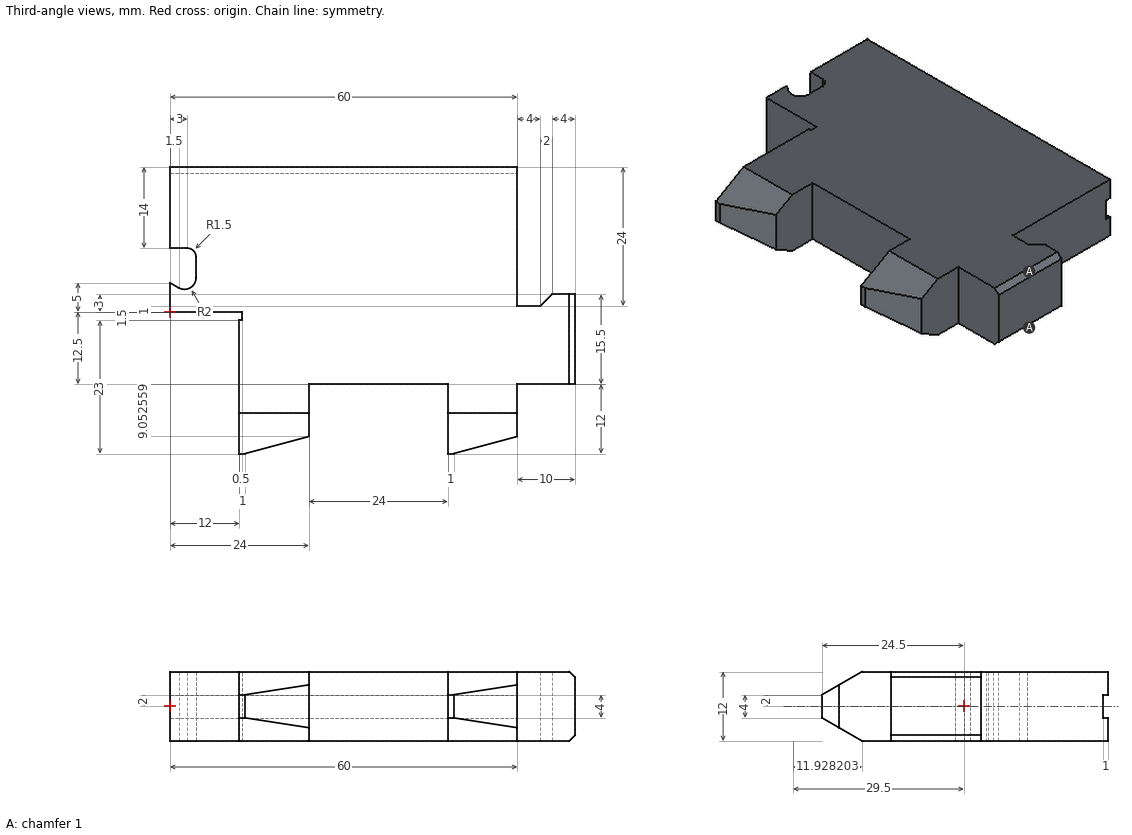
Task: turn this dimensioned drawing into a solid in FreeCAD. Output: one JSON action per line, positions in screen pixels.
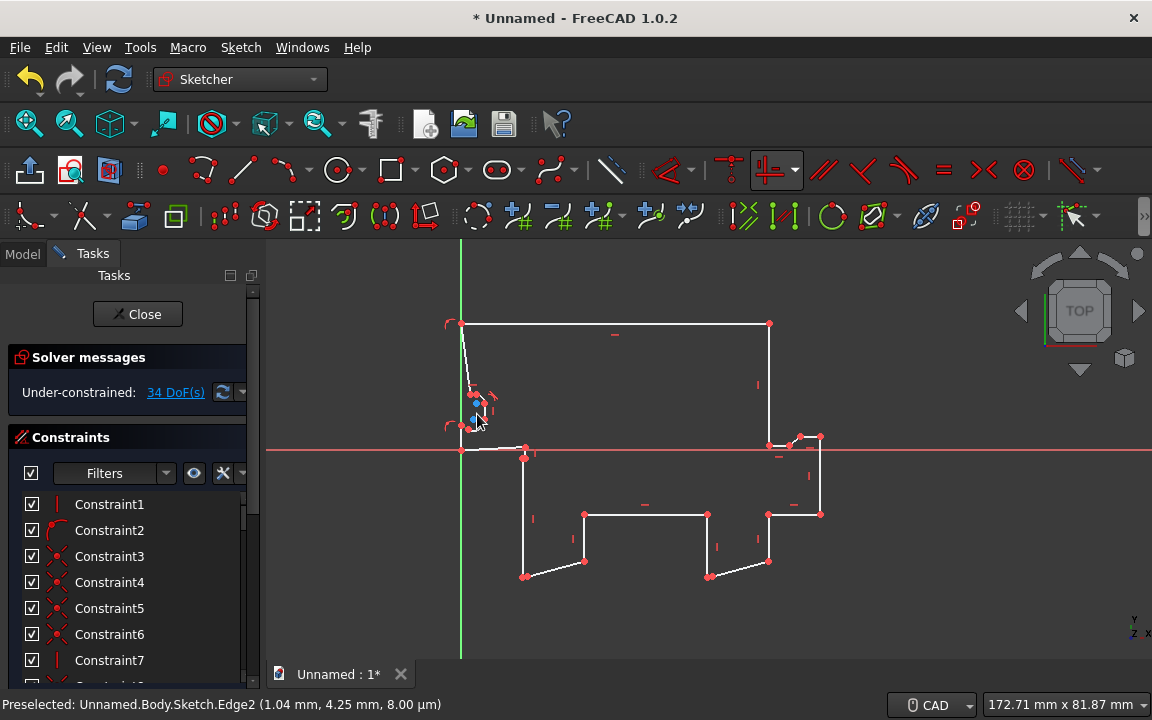
{"action": "scroll", "coordinate": [475, 431], "scroll_direction": "up", "scroll_amount": 4}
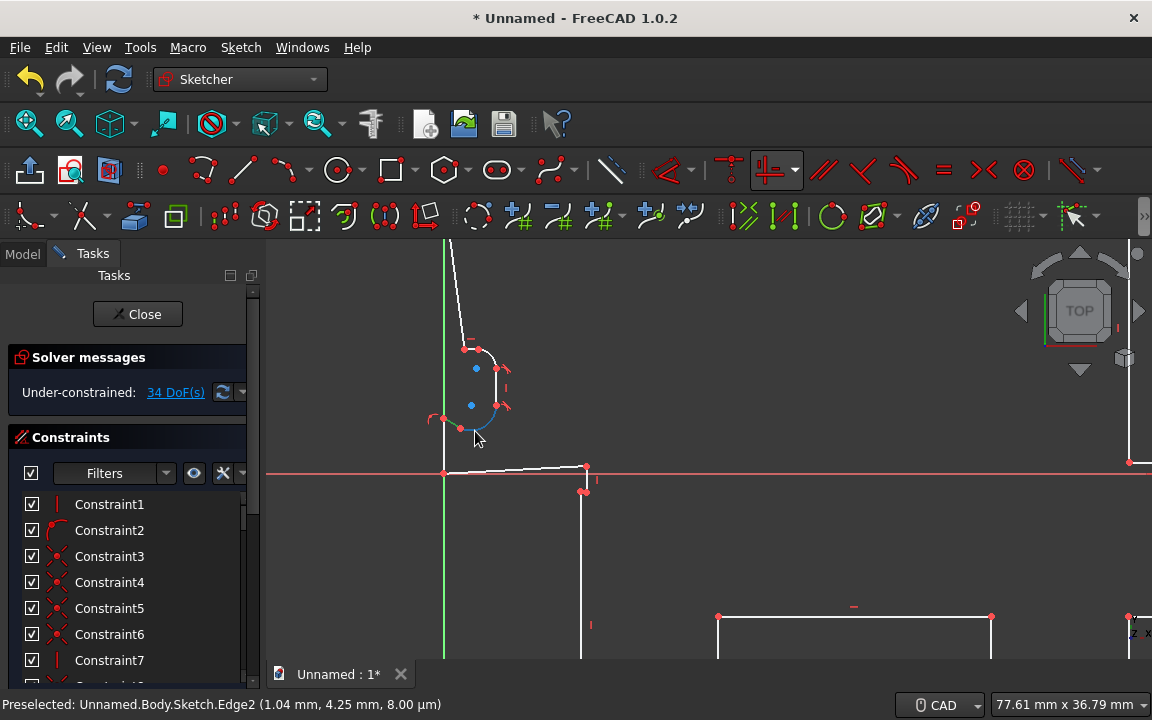
{"action": "left_click", "coordinate": [475, 430]}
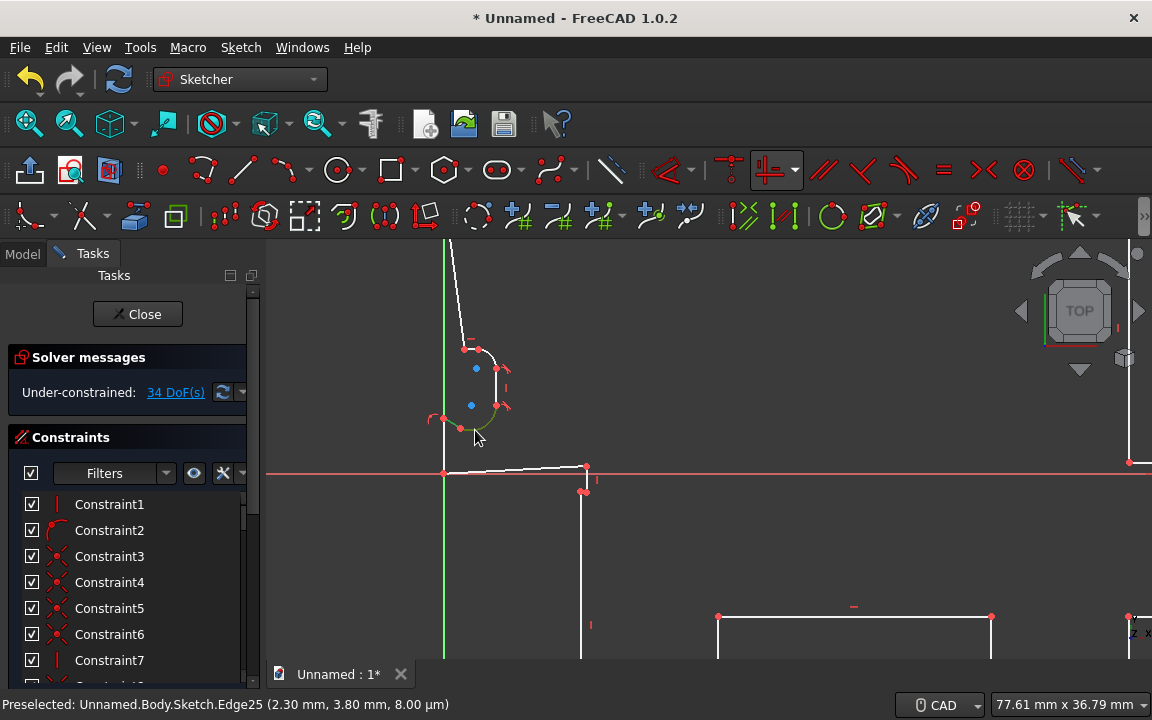
{"action": "left_click", "coordinate": [904, 170]}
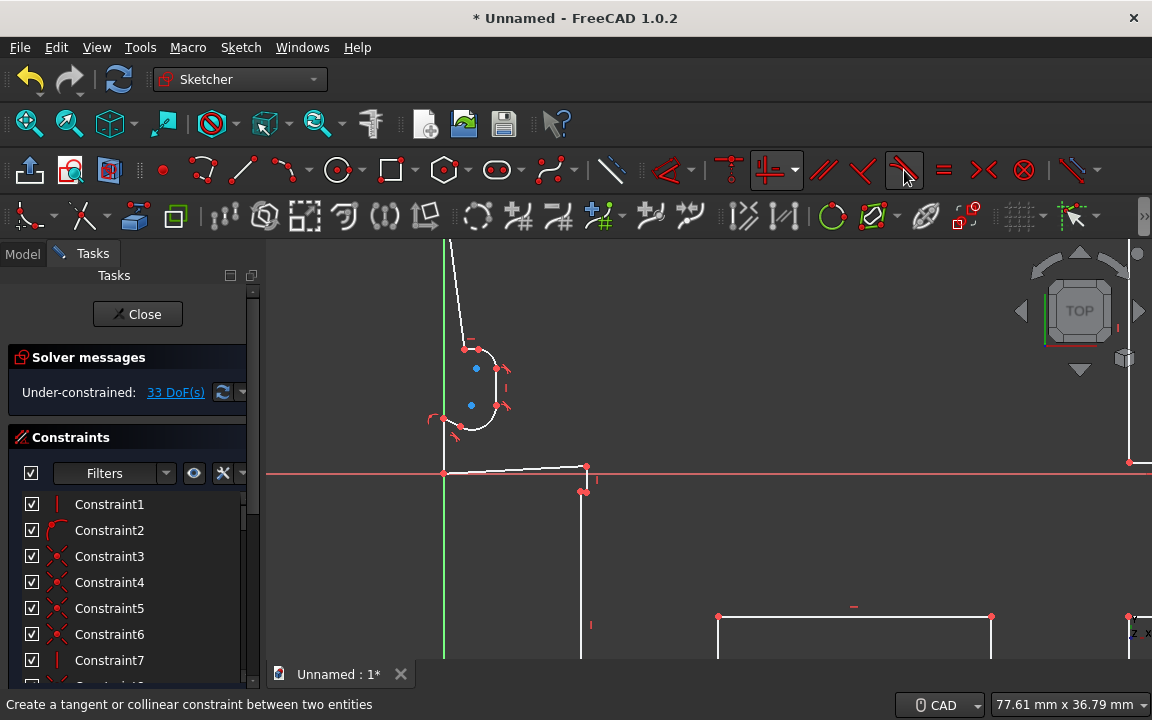
{"action": "scroll", "coordinate": [471, 349], "scroll_direction": "up", "scroll_amount": 4}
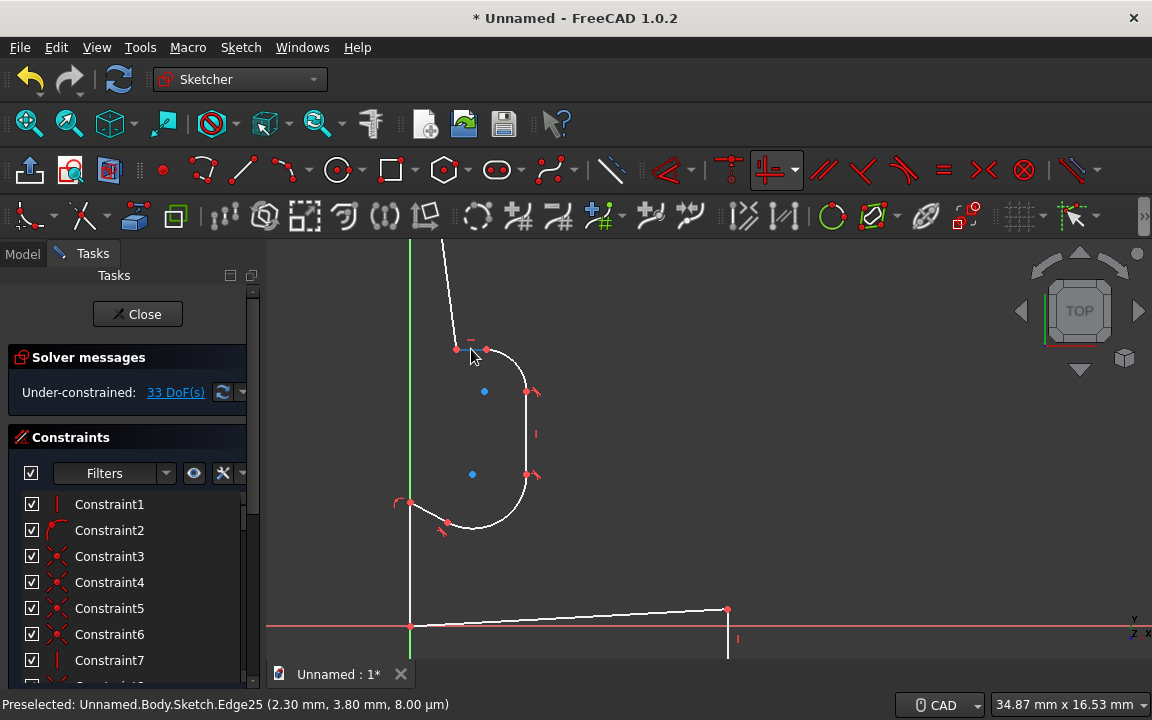
{"action": "left_click", "coordinate": [471, 350]}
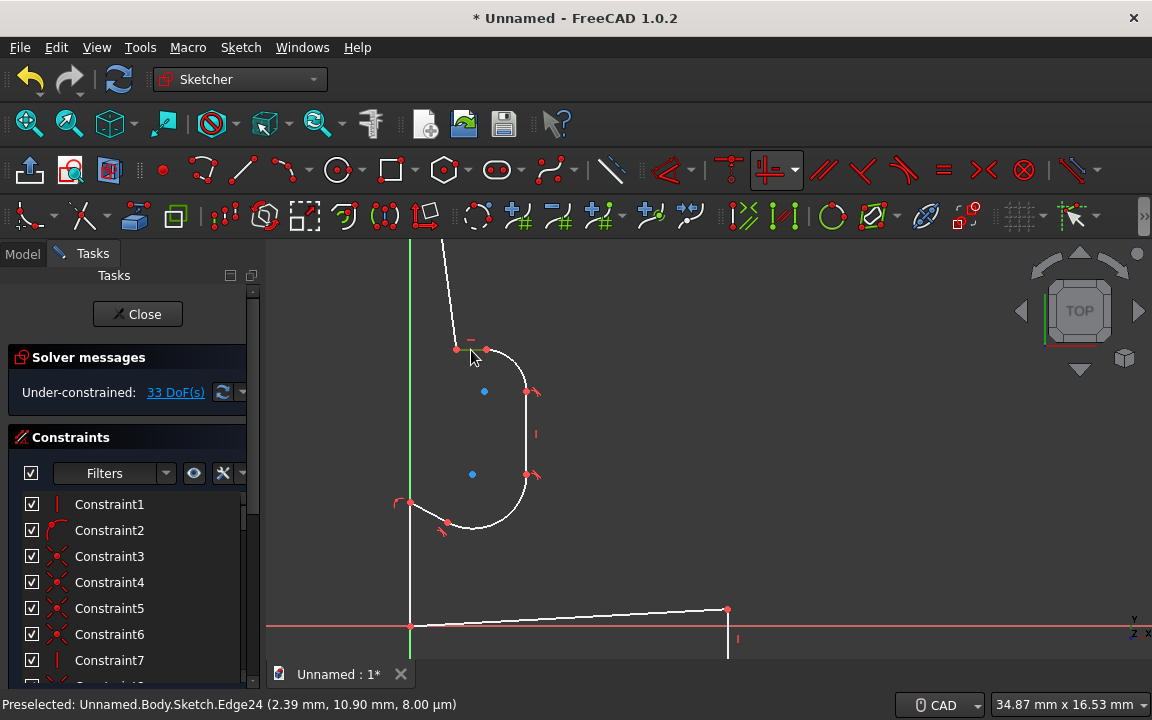
{"action": "left_click", "coordinate": [522, 373]}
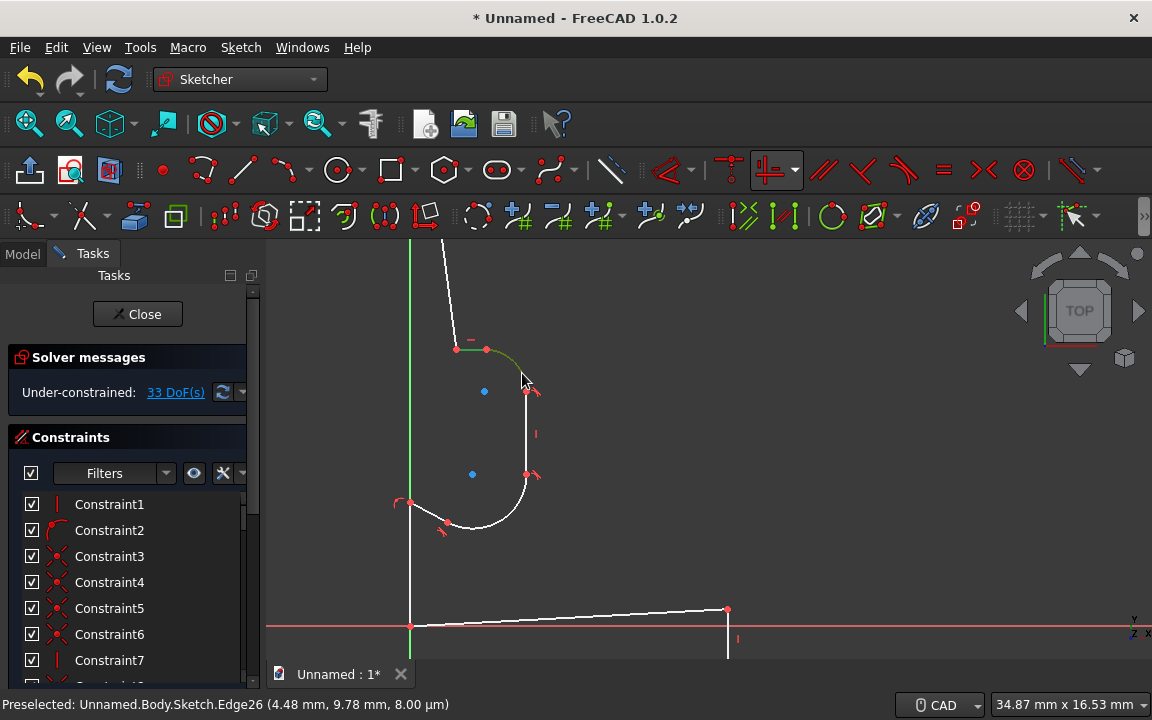
{"action": "left_click", "coordinate": [904, 170]}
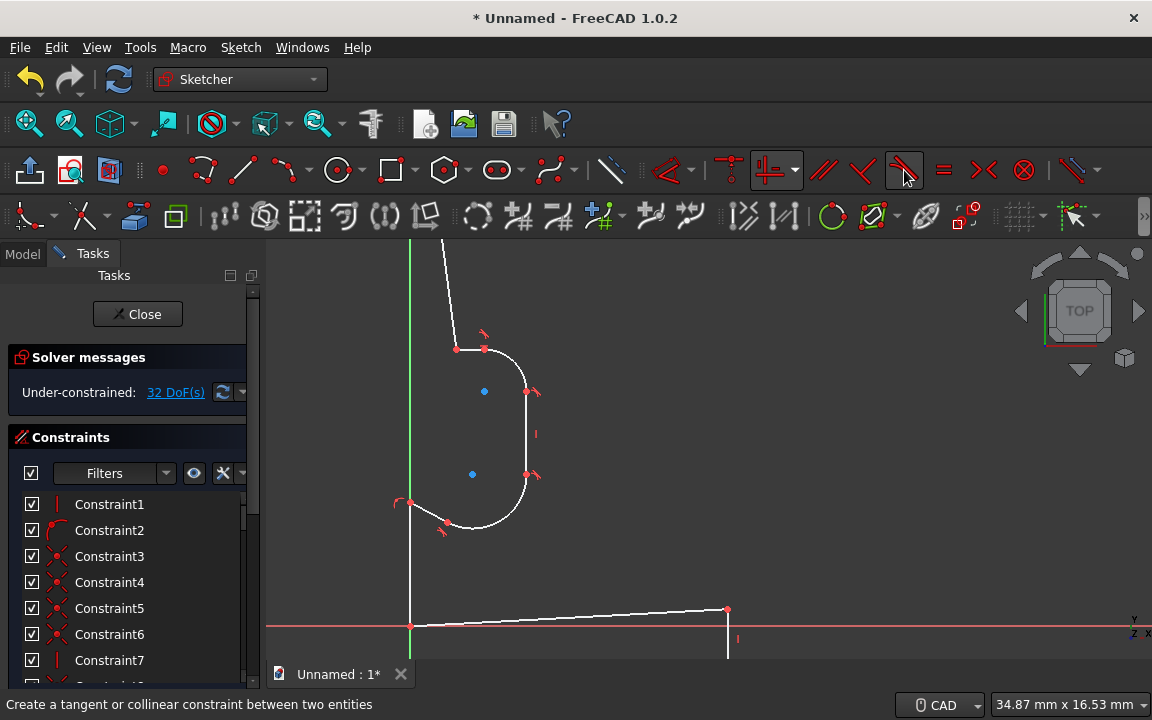
{"action": "left_click", "coordinate": [633, 614]}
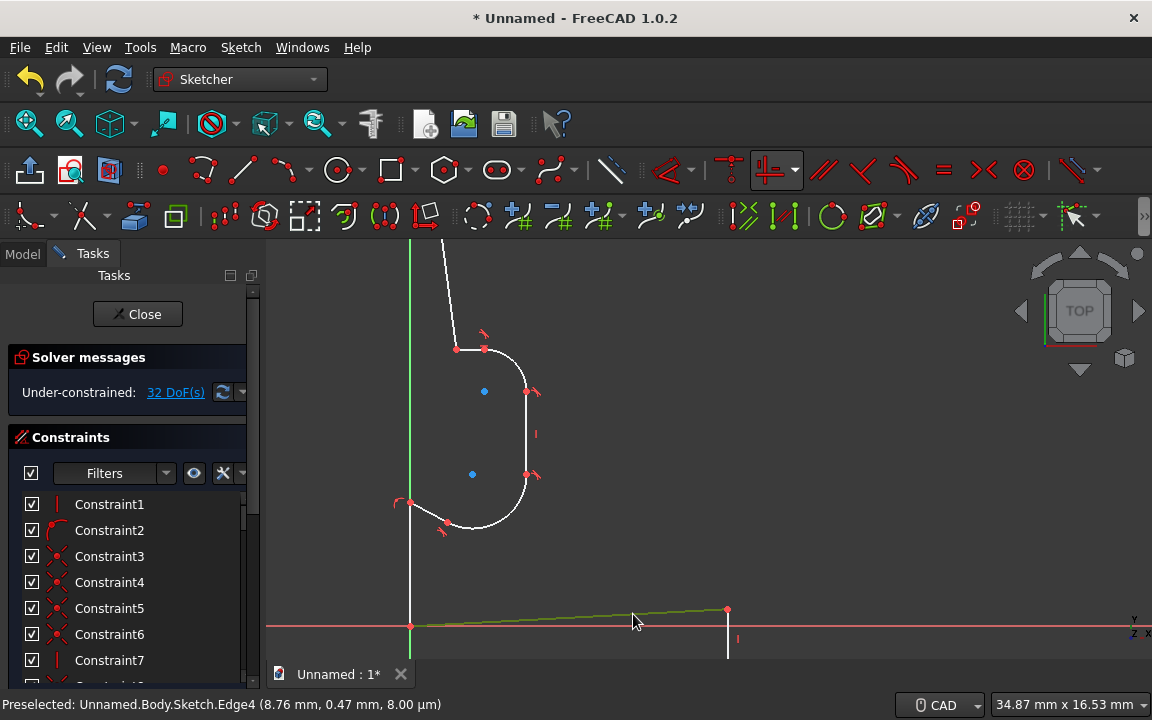
{"action": "key", "text": "h"}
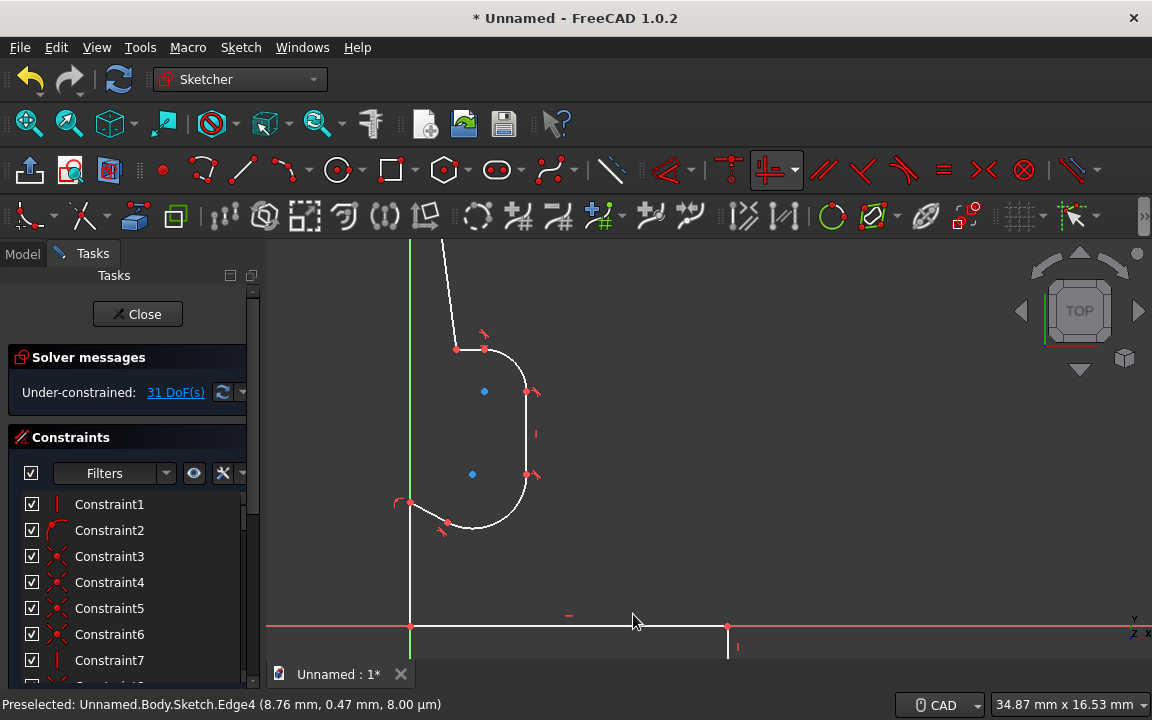
{"action": "scroll", "coordinate": [474, 406], "scroll_direction": "down", "scroll_amount": 8}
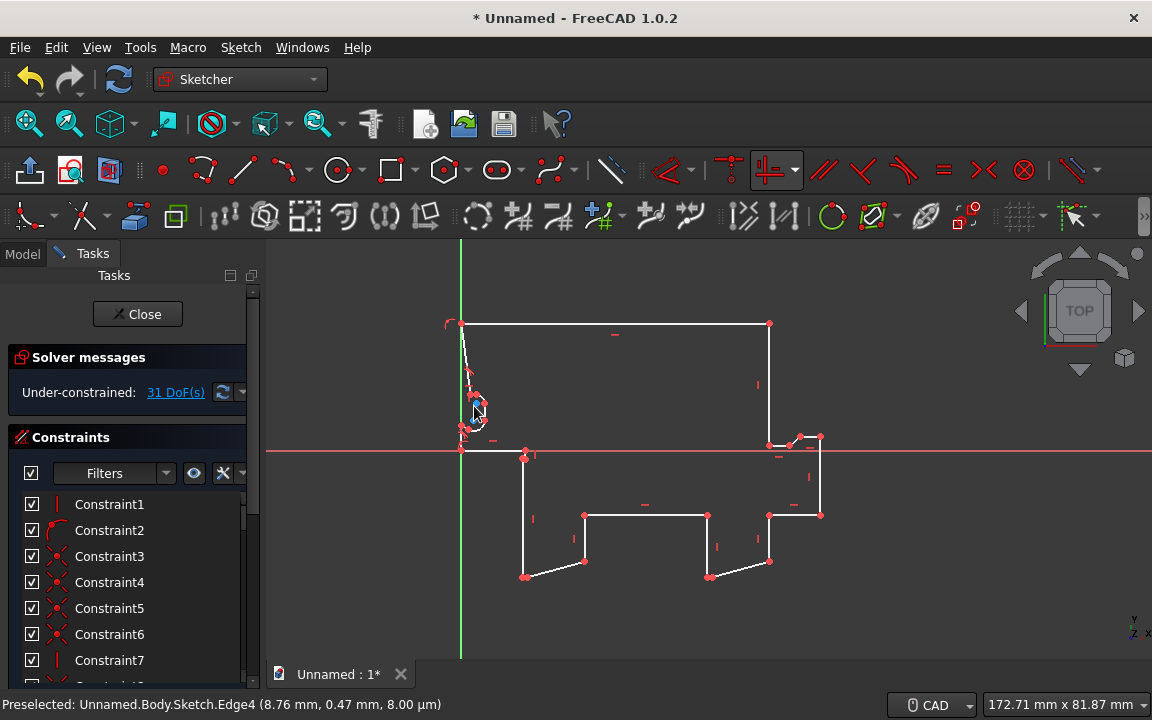
{"action": "scroll", "coordinate": [524, 459], "scroll_direction": "up", "scroll_amount": 12}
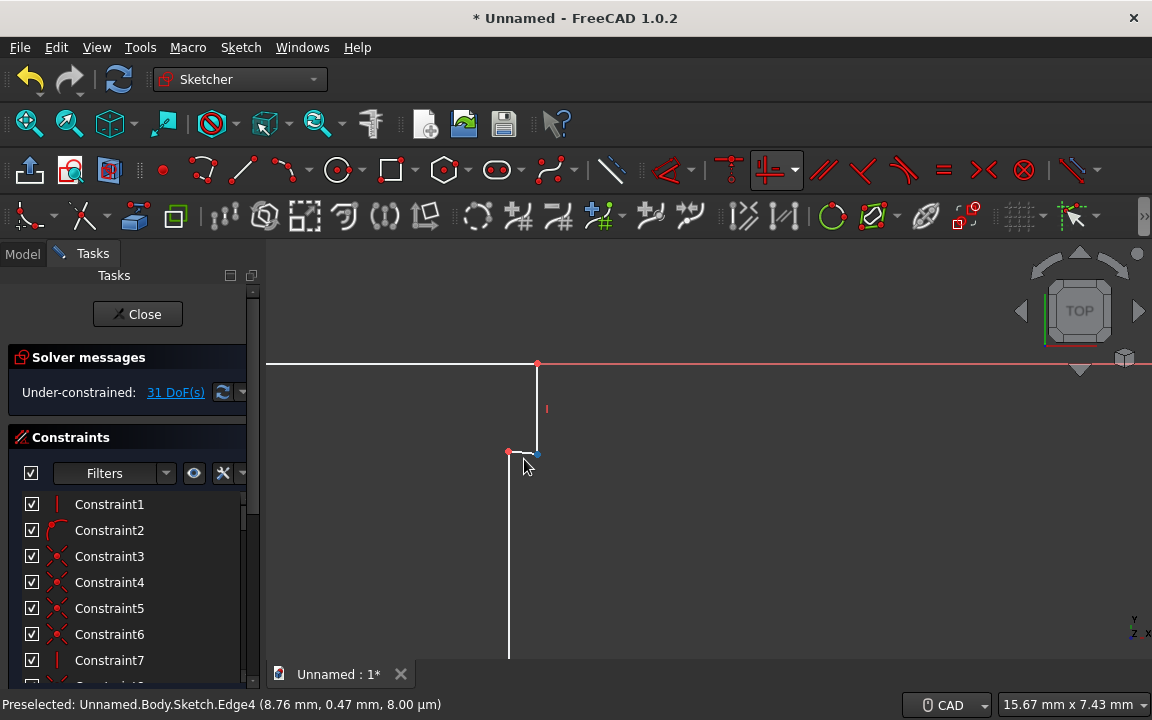
{"action": "left_click", "coordinate": [523, 453]}